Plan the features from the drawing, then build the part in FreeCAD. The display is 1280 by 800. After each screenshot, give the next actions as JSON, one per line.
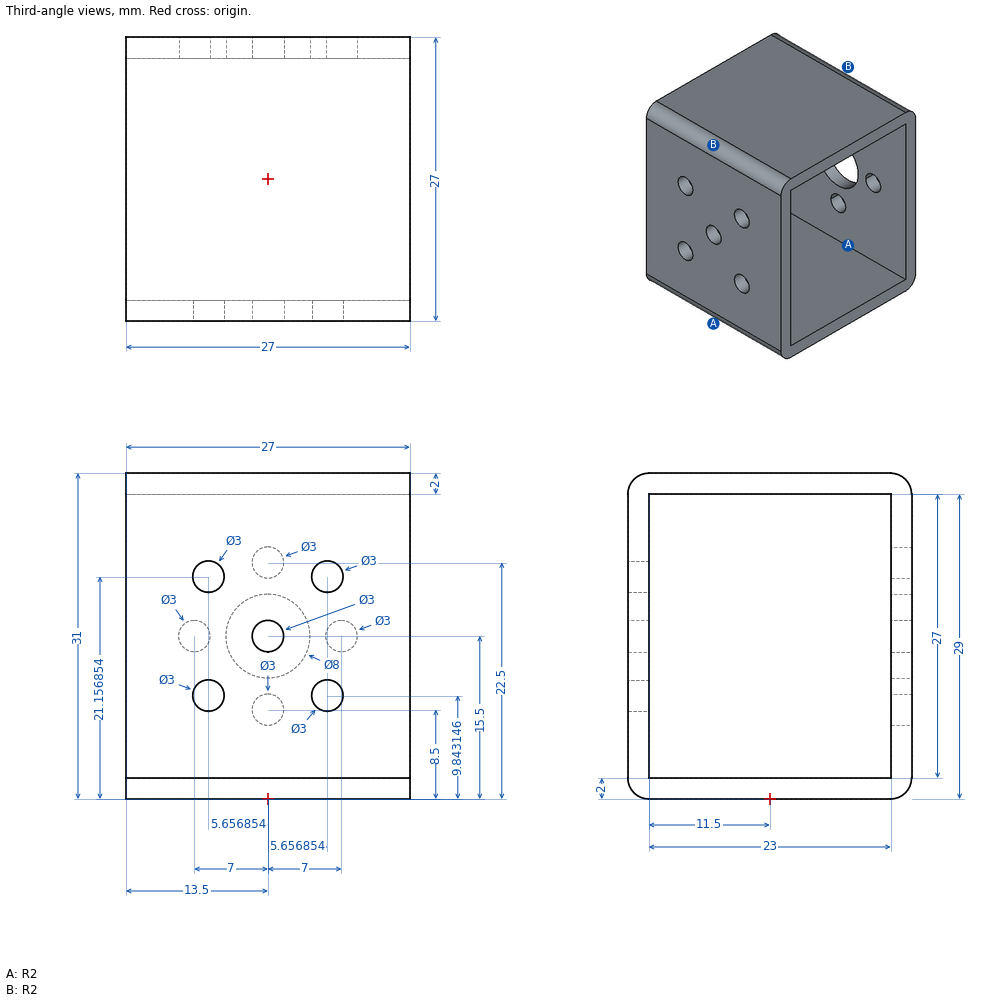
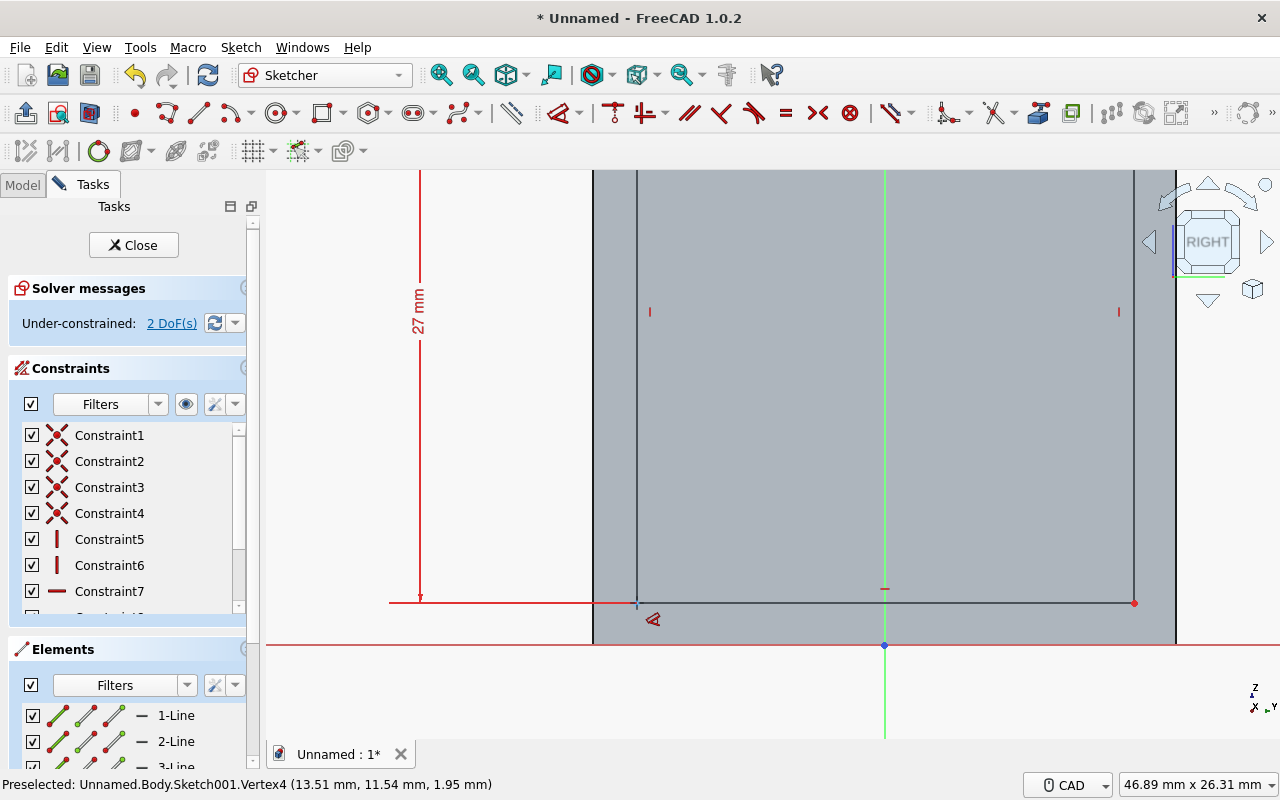
{"action": "left_click", "coordinate": [637, 603]}
{"action": "left_click", "coordinate": [603, 624]}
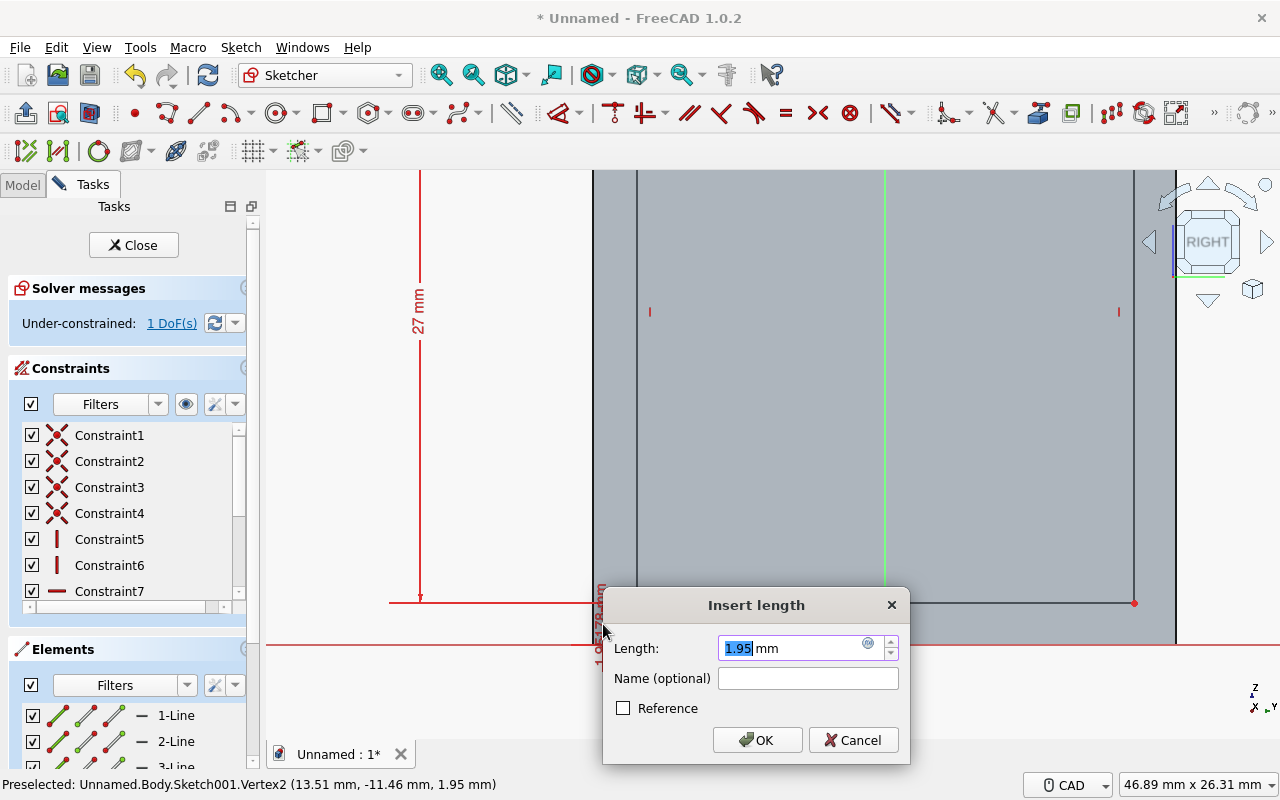
{"action": "type", "text": "2"}
{"action": "key", "text": "Return"}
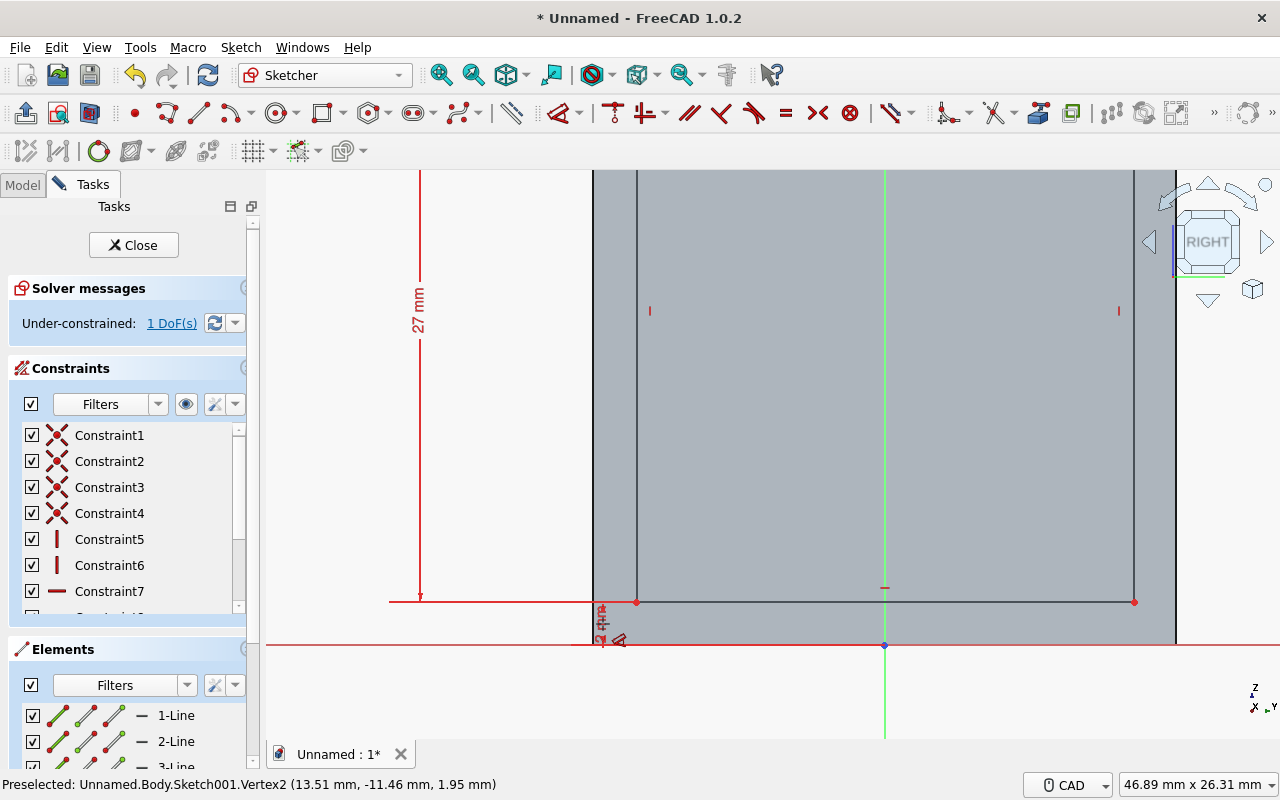
{"action": "scroll", "coordinate": [486, 604], "scroll_direction": "down", "scroll_amount": 3}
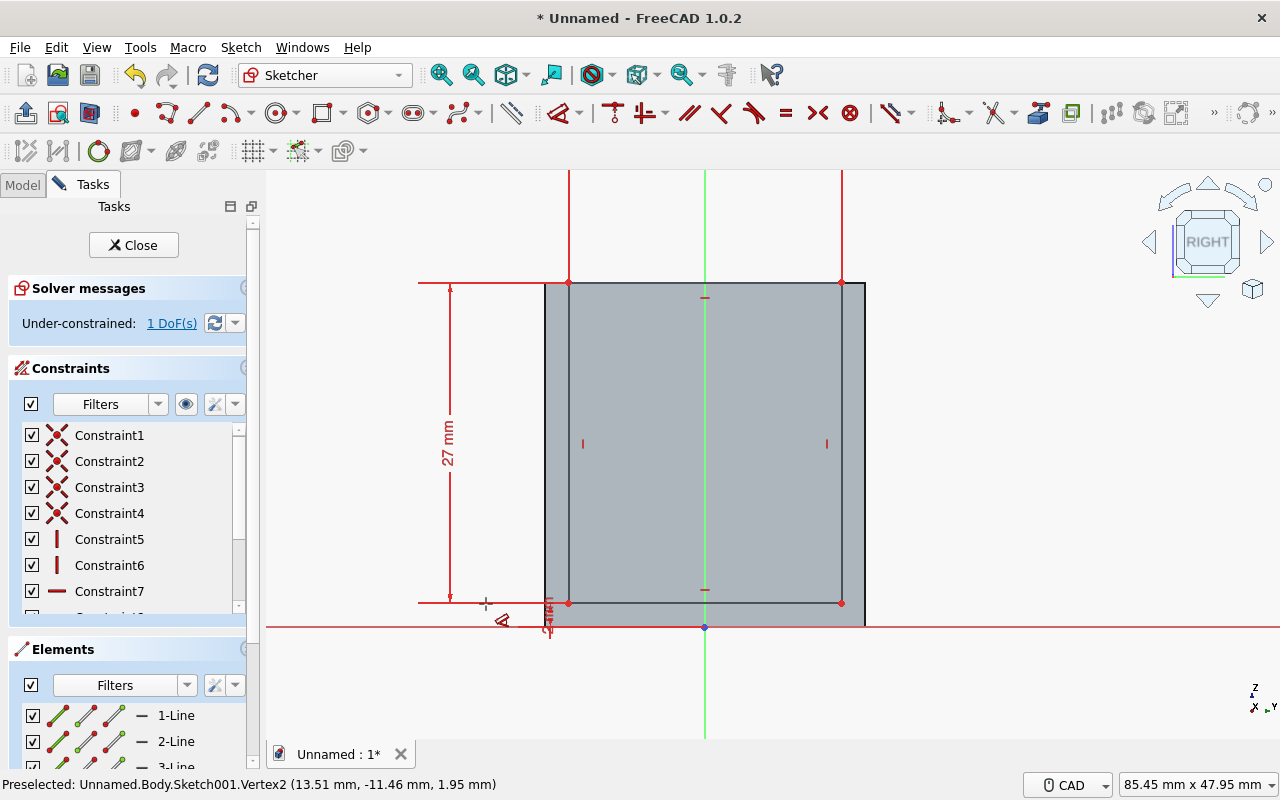
{"action": "left_click", "coordinate": [569, 283]}
{"action": "left_click", "coordinate": [637, 661]}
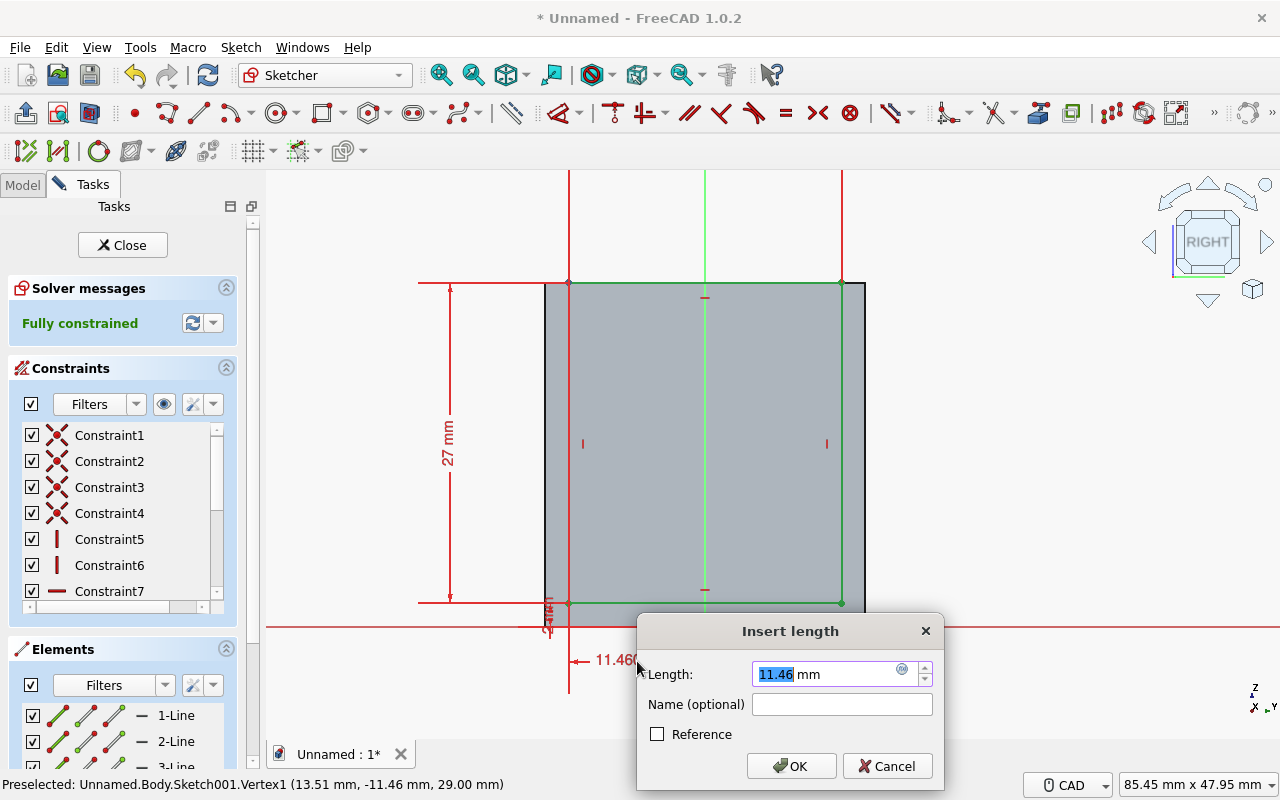
{"action": "type", "text": "11.5"}
{"action": "key", "text": "Return"}
{"action": "key", "text": "Escape"}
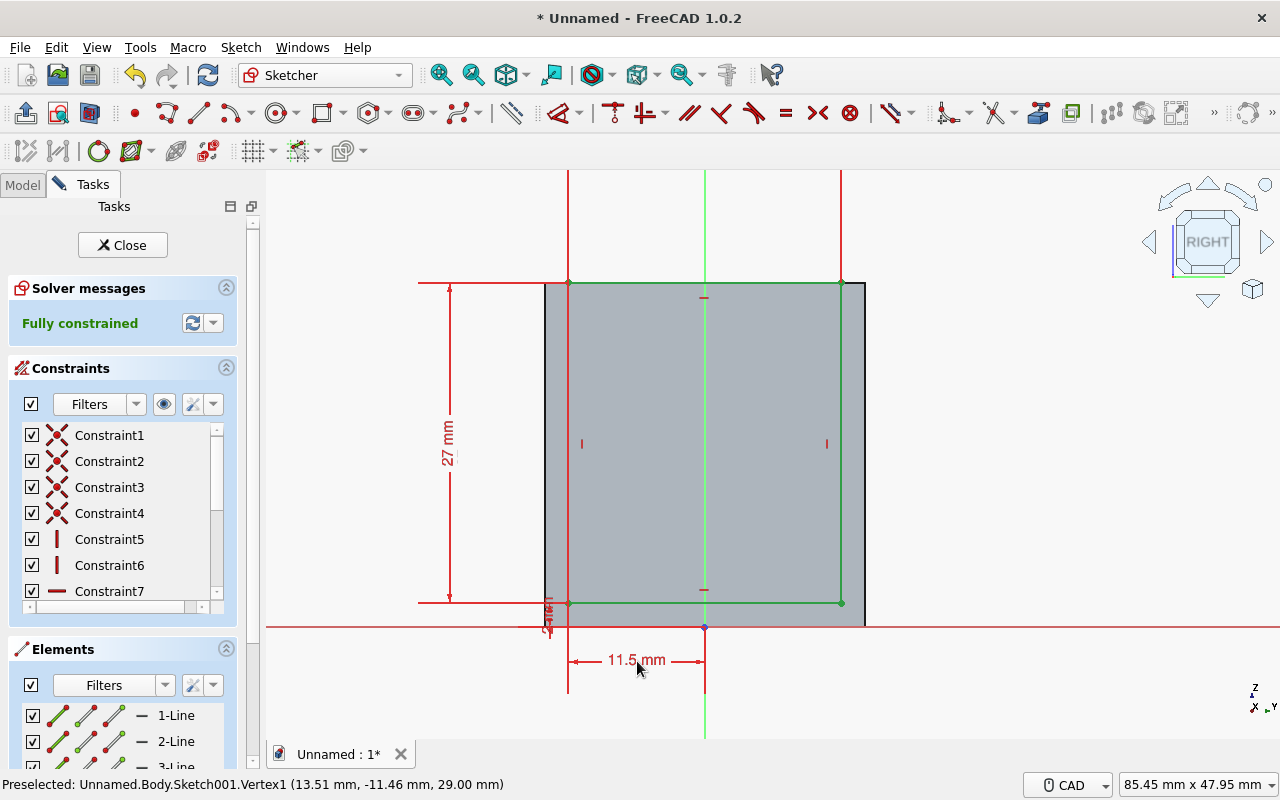
{"action": "left_click", "coordinate": [123, 245]}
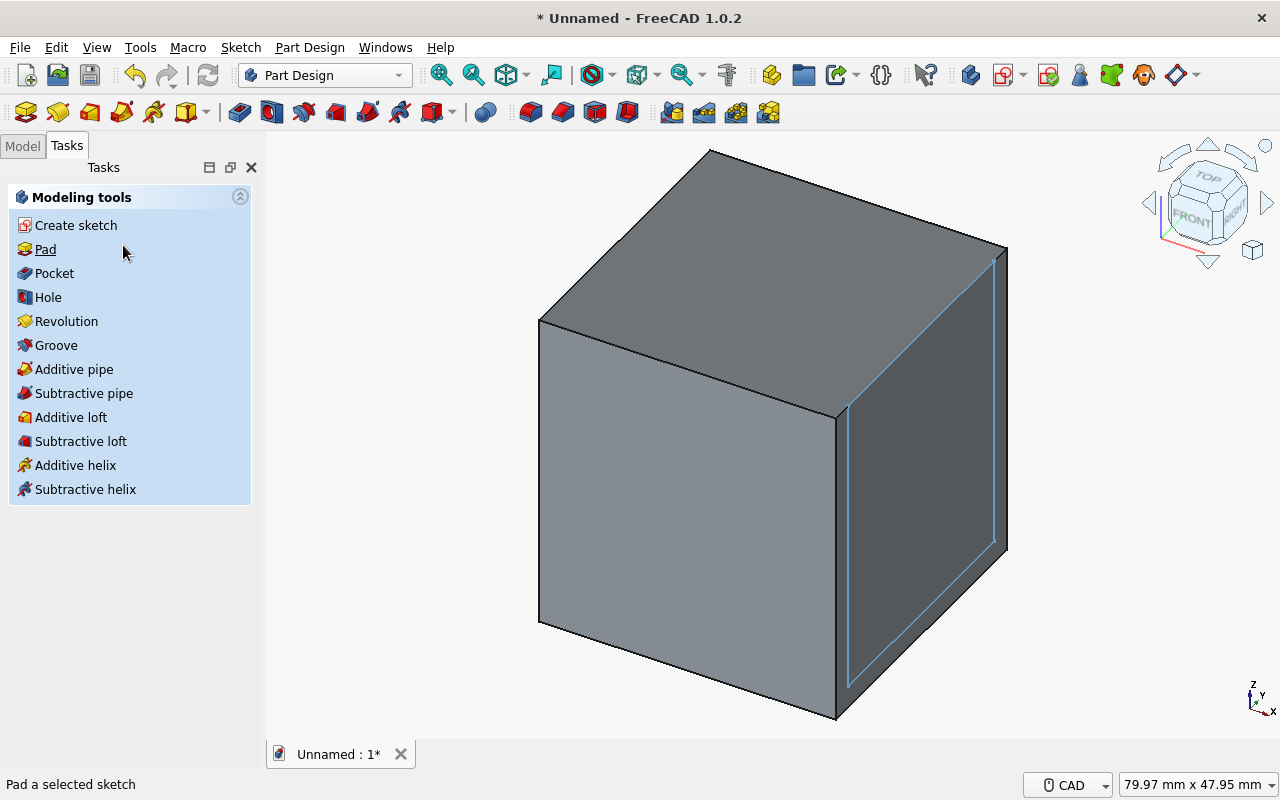
{"action": "left_click", "coordinate": [240, 112]}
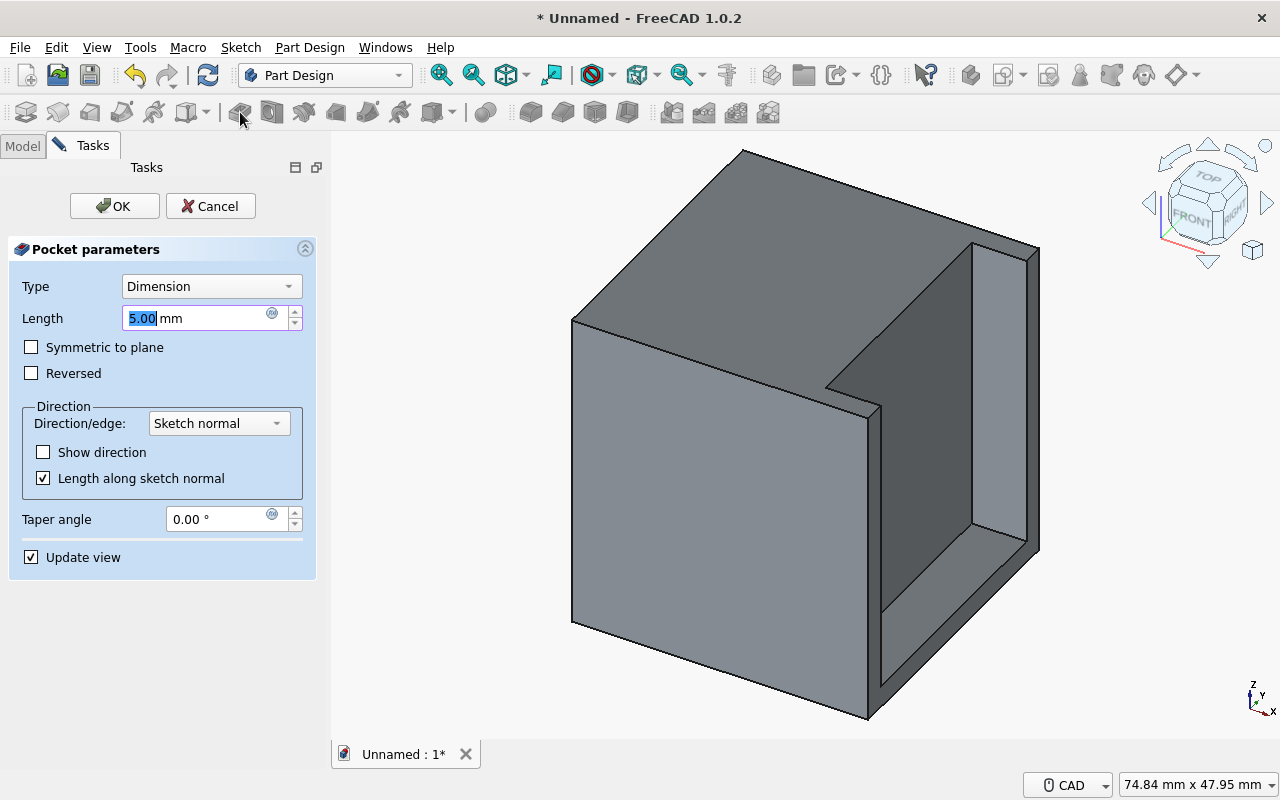
{"action": "type", "text": "27"}
{"action": "key", "text": "Tab"}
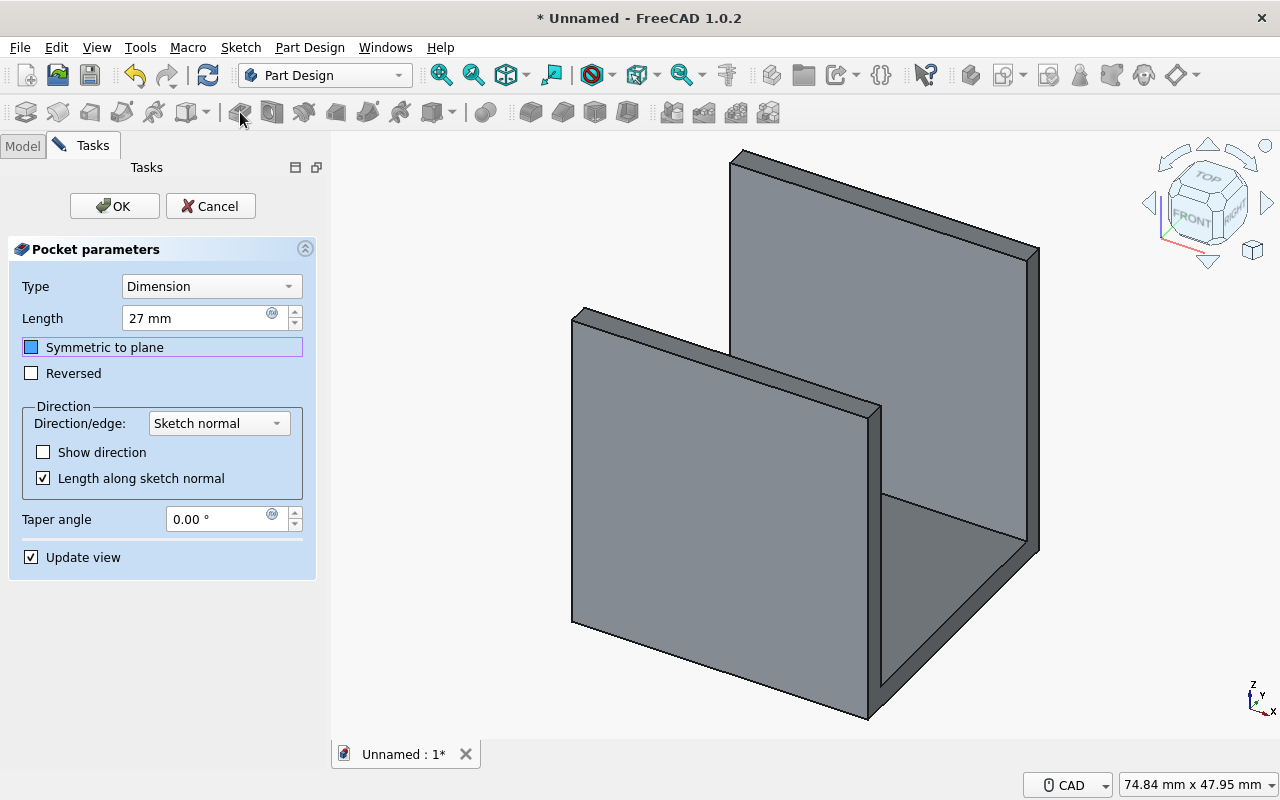
{"action": "left_click", "coordinate": [115, 206]}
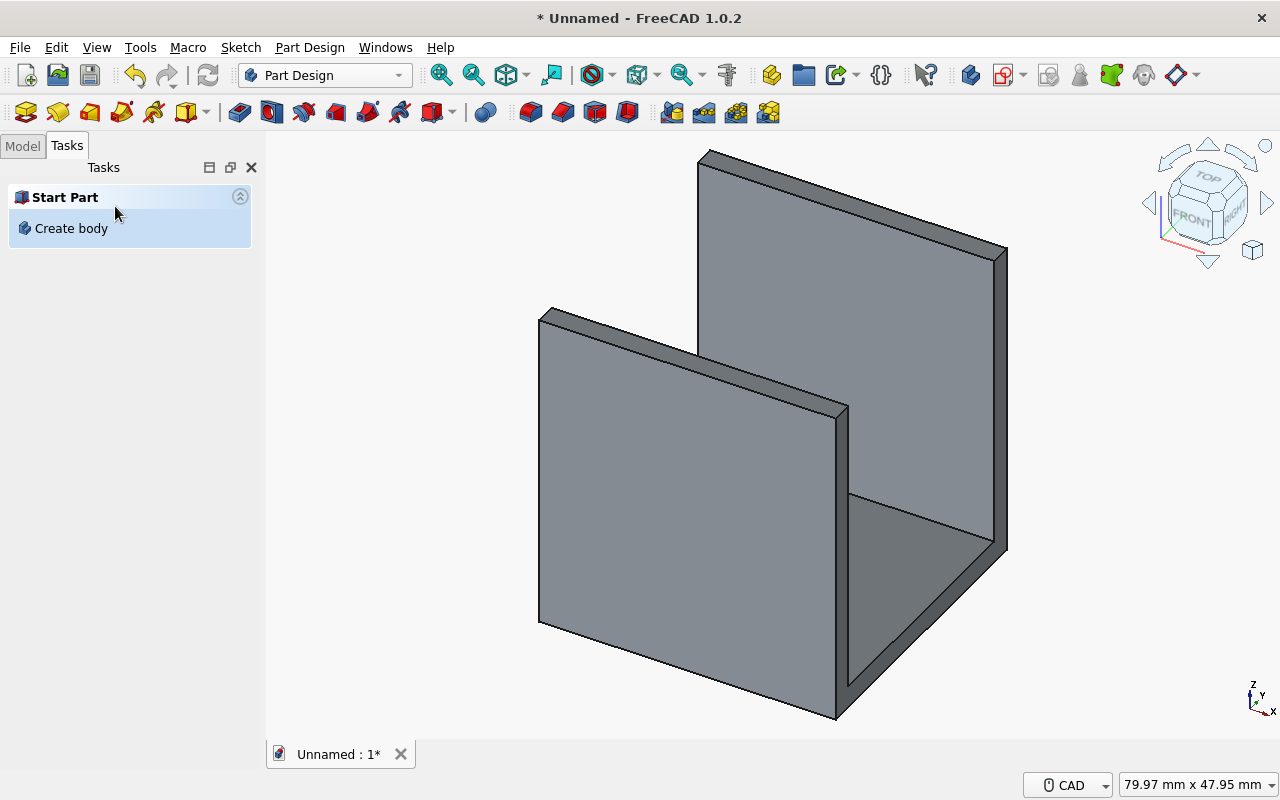
{"action": "key", "text": "4"}